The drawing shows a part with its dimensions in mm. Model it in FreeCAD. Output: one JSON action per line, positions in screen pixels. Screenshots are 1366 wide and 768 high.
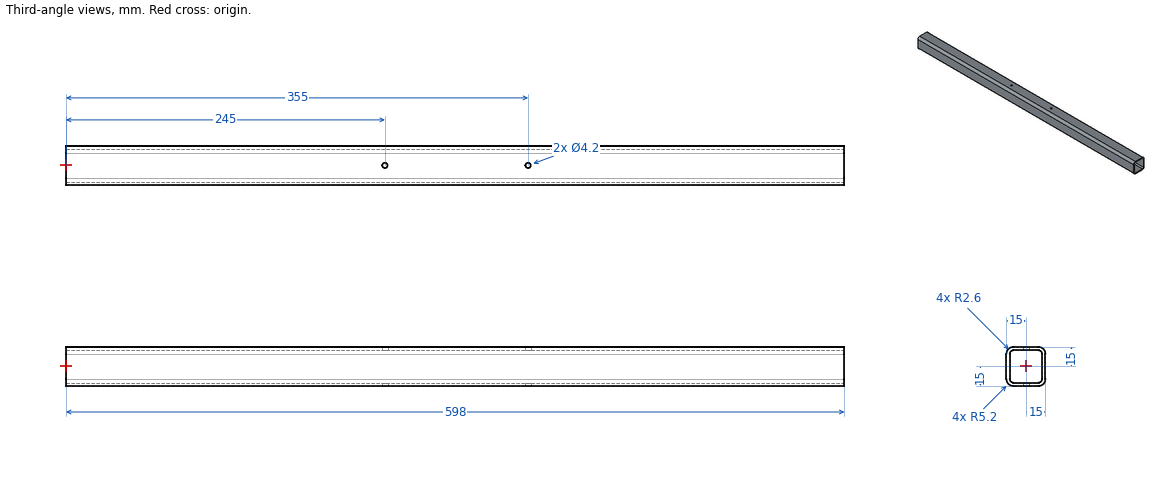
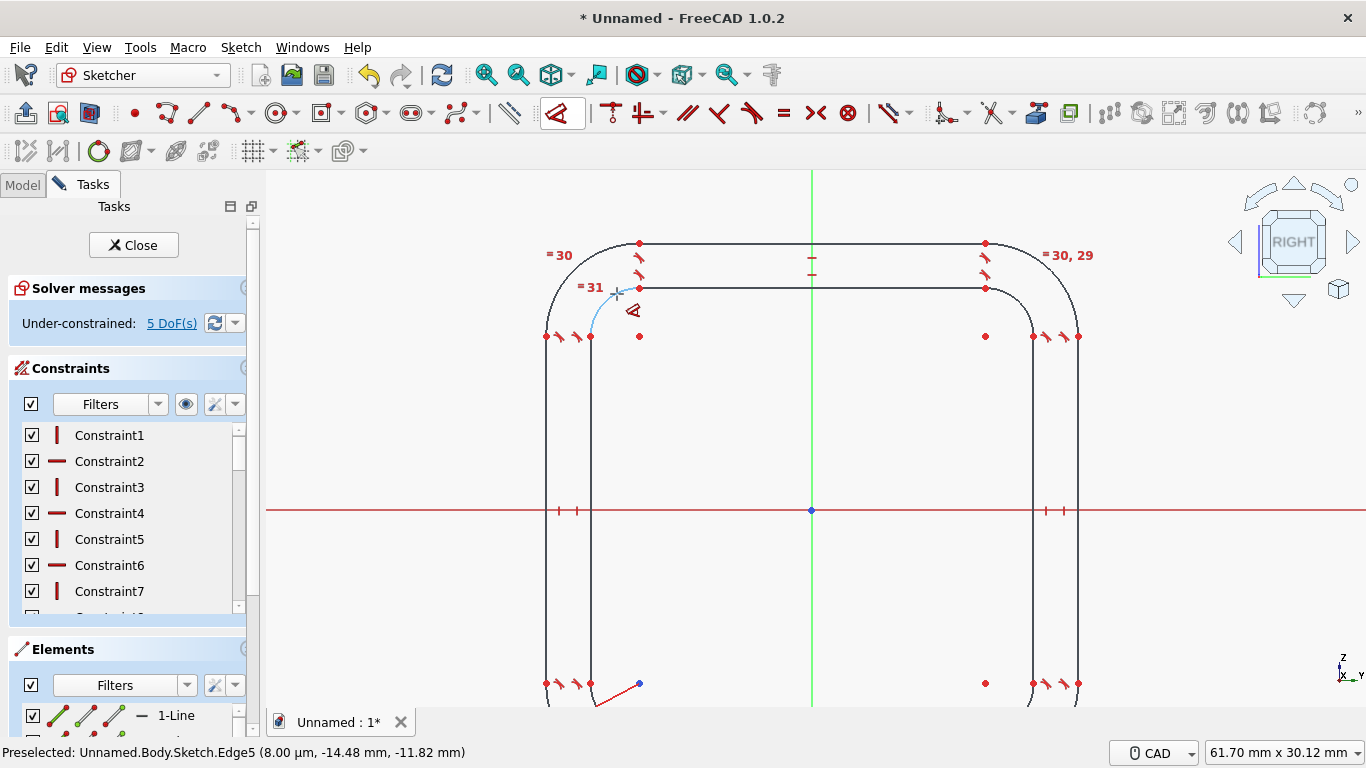
{"action": "left_click", "coordinate": [617, 293]}
{"action": "left_click", "coordinate": [680, 267]}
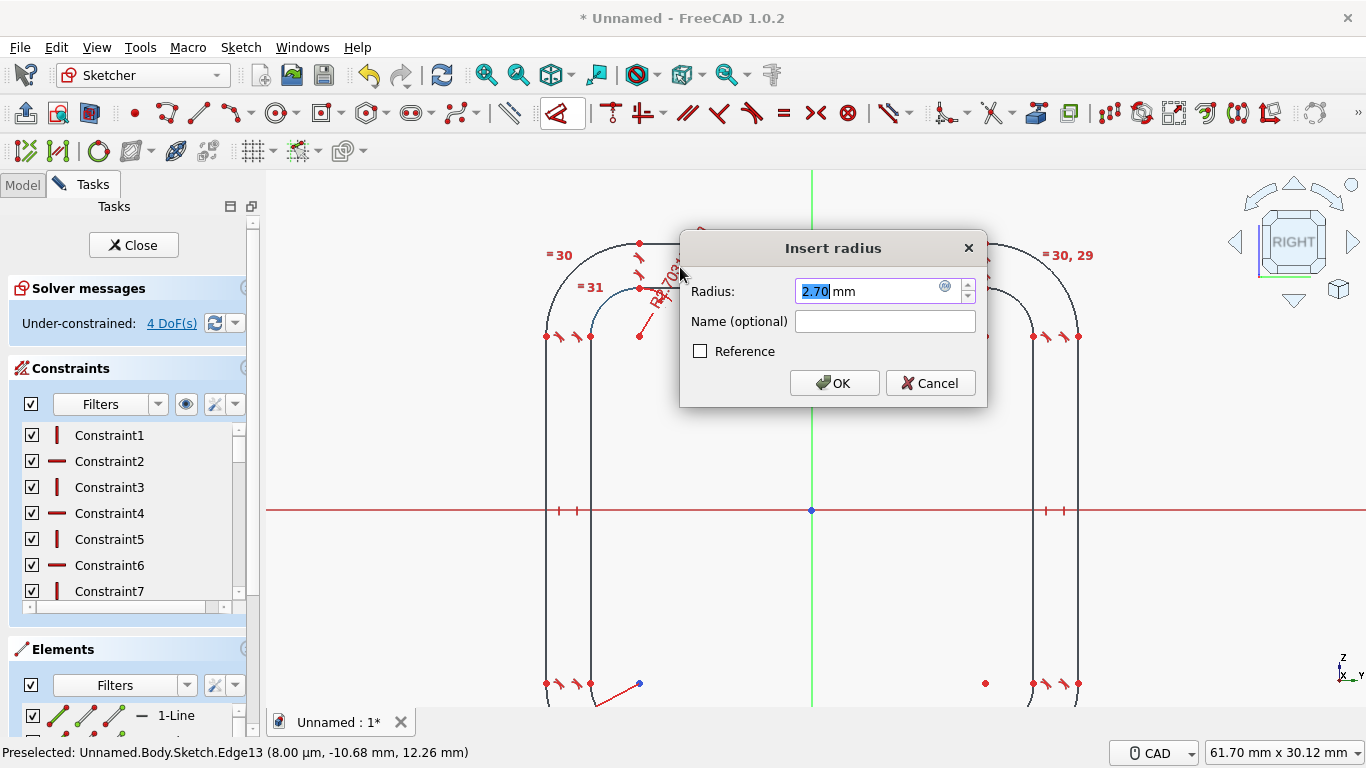
{"action": "type", "text": "2.6"}
{"action": "key", "text": "Return"}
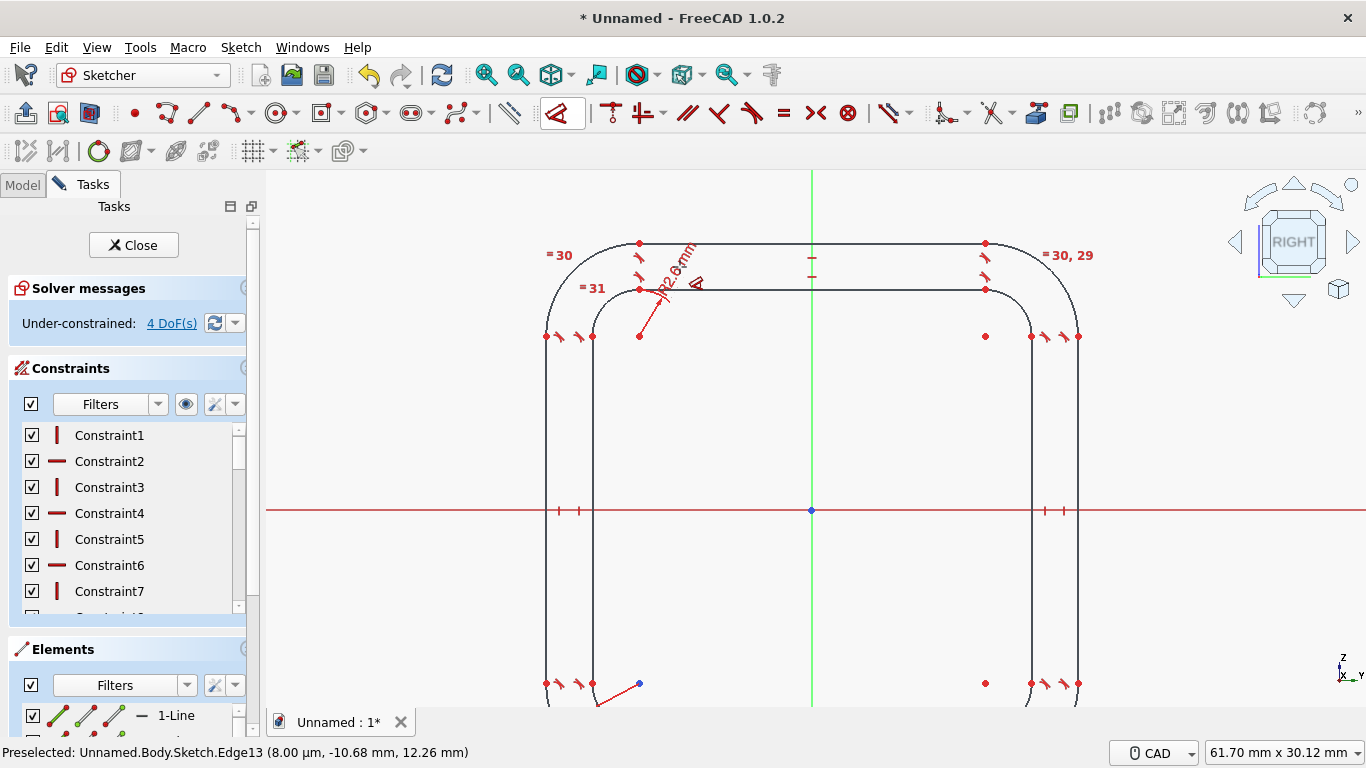
{"action": "left_click", "coordinate": [546, 336]}
{"action": "left_click", "coordinate": [586, 302]}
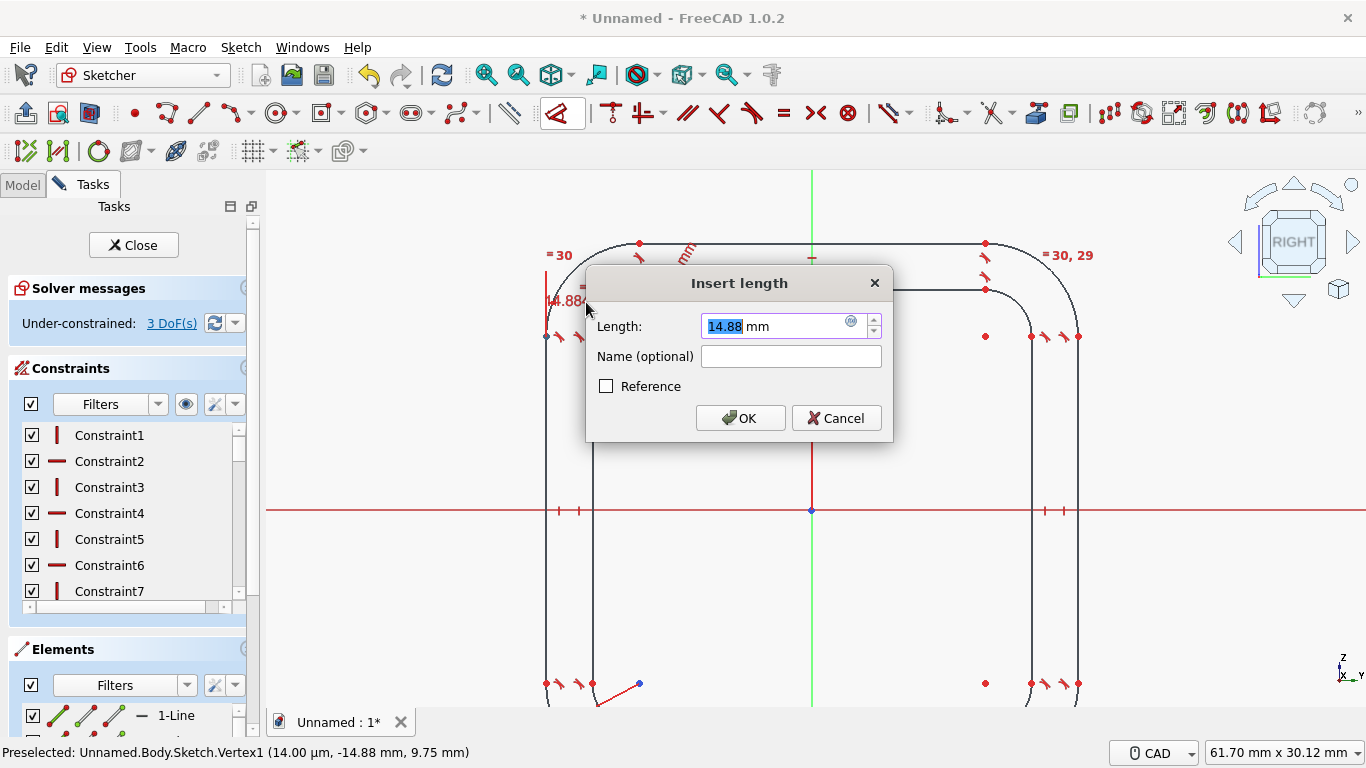
{"action": "type", "text": "15"}
{"action": "key", "text": "Return"}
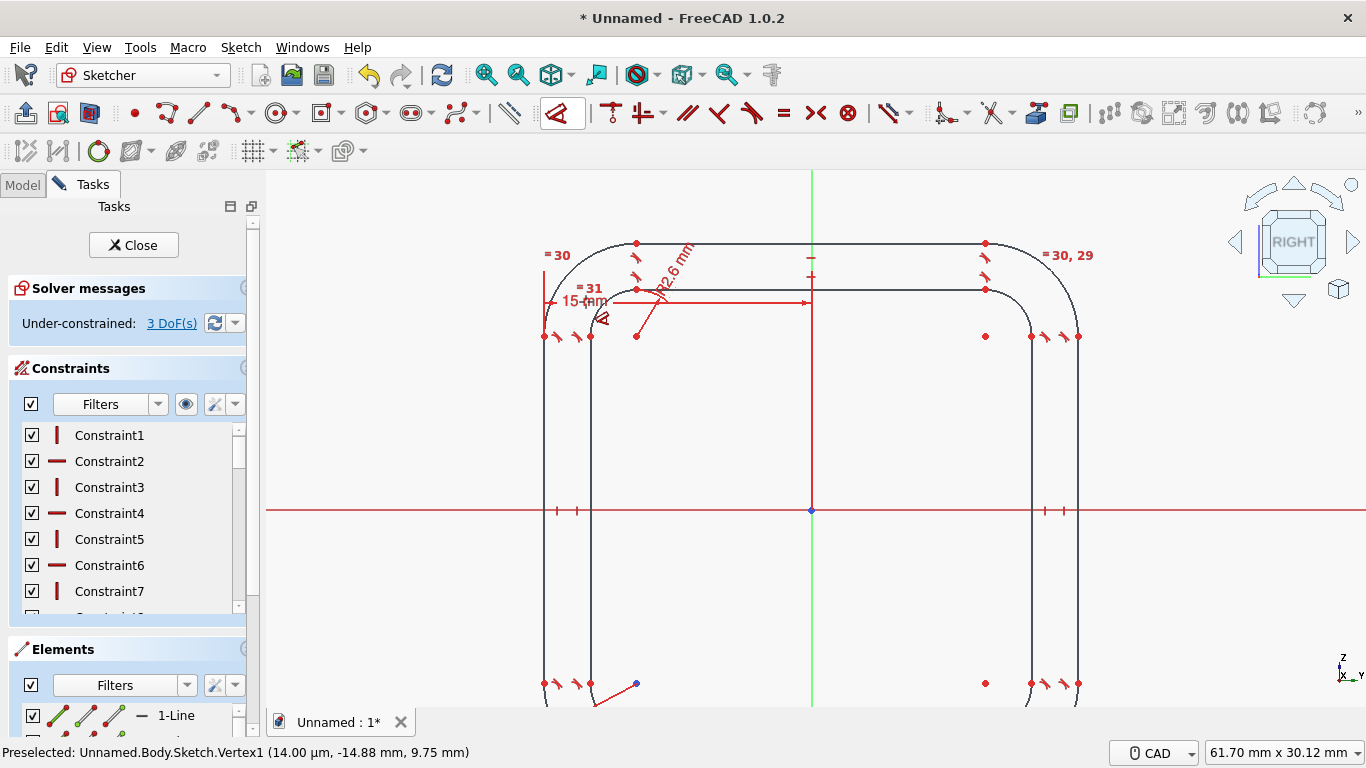
{"action": "scroll", "coordinate": [617, 293], "scroll_direction": "down", "scroll_amount": 2}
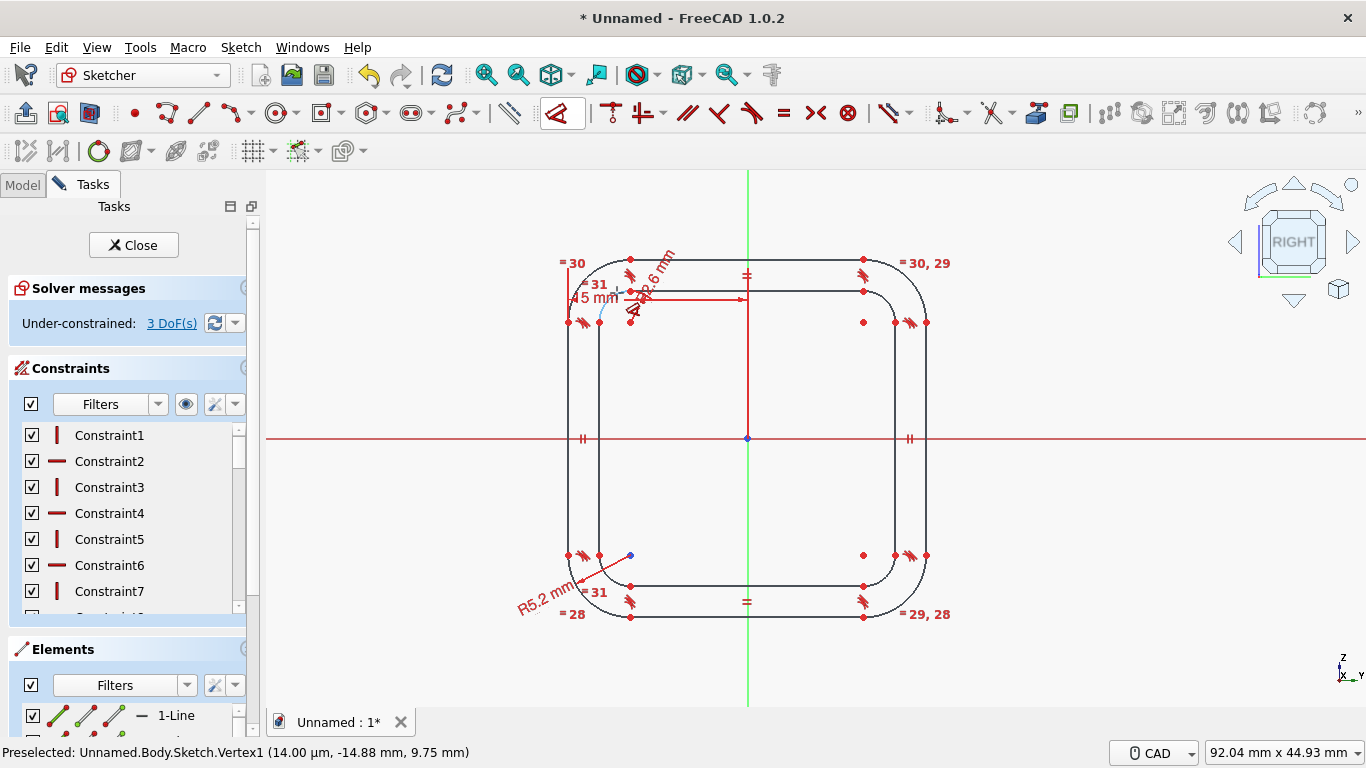
{"action": "left_click", "coordinate": [630, 617]}
{"action": "left_click", "coordinate": [782, 528]}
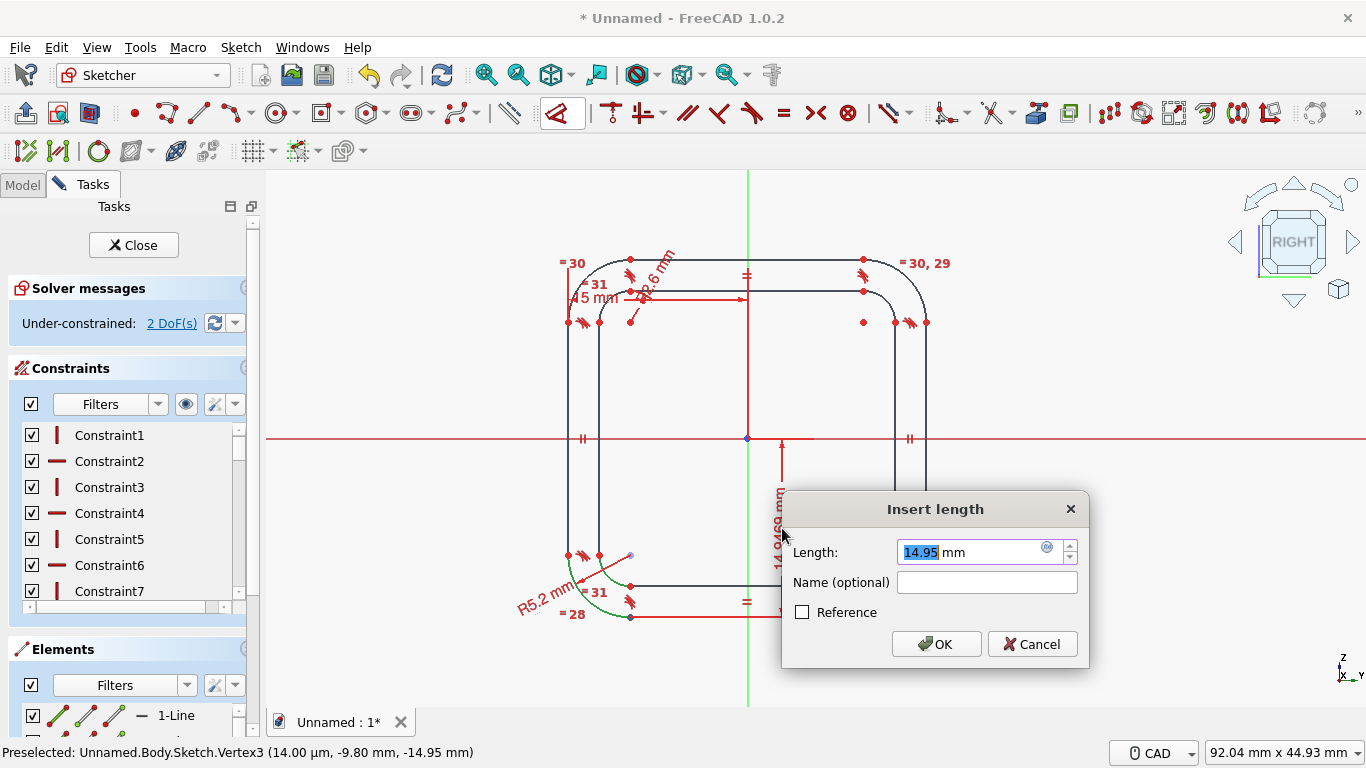
{"action": "type", "text": "15"}
{"action": "key", "text": "Return"}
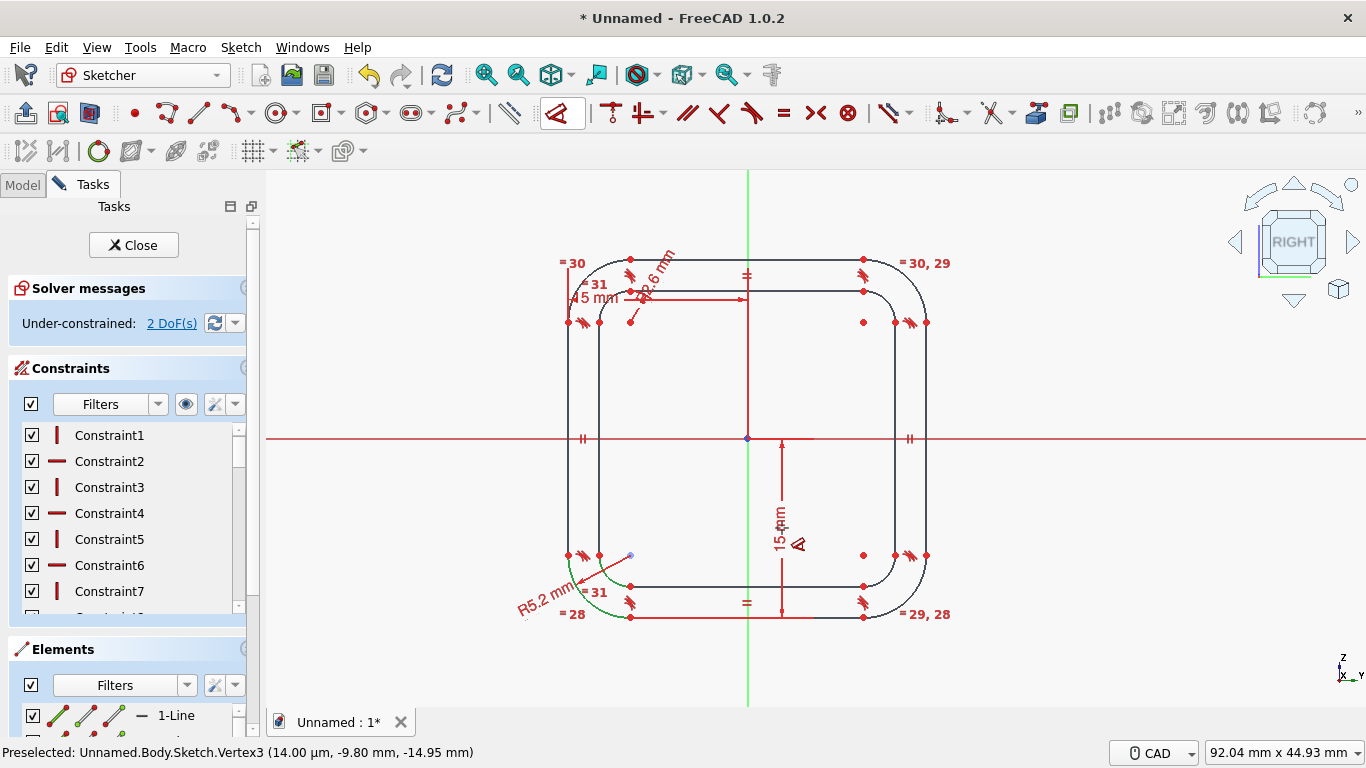
{"action": "left_click", "coordinate": [926, 556]}
{"action": "left_click", "coordinate": [899, 590]}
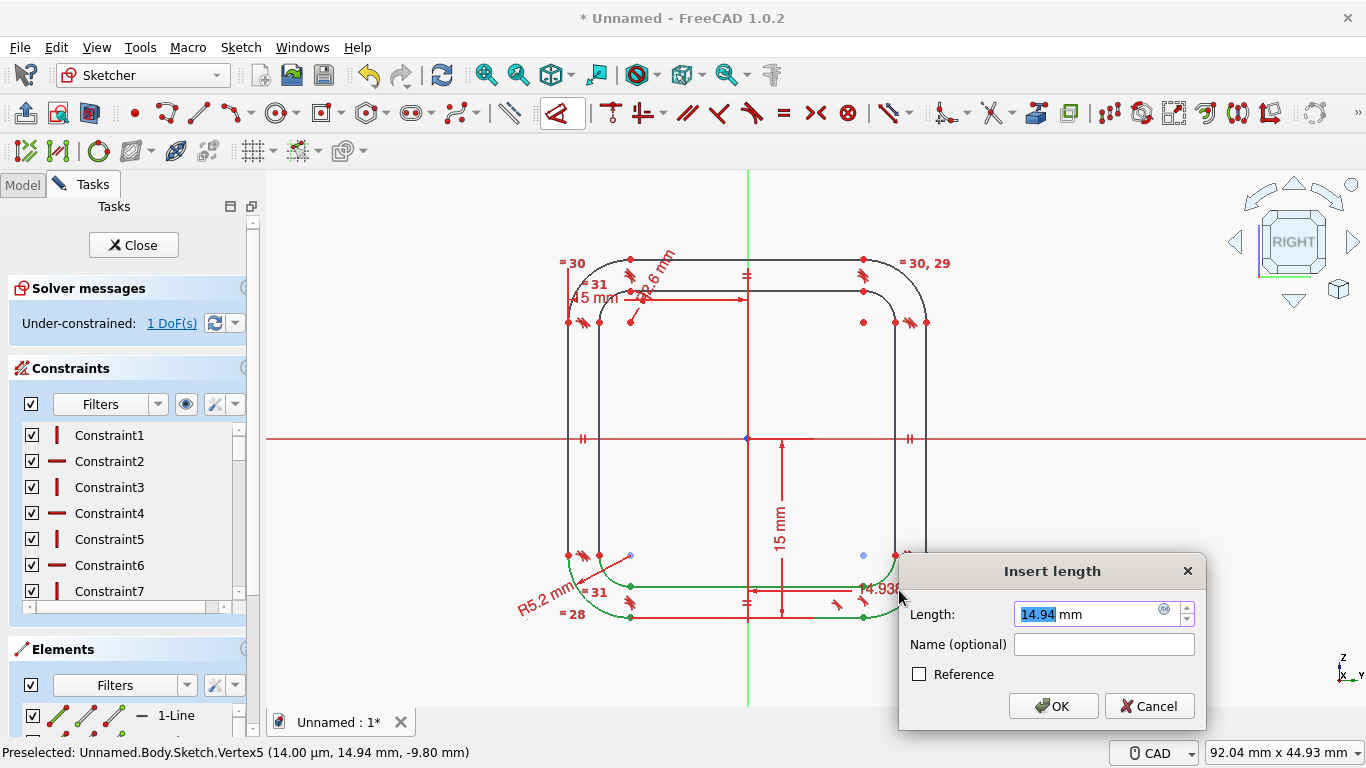
{"action": "type", "text": "15"}
{"action": "key", "text": "Return"}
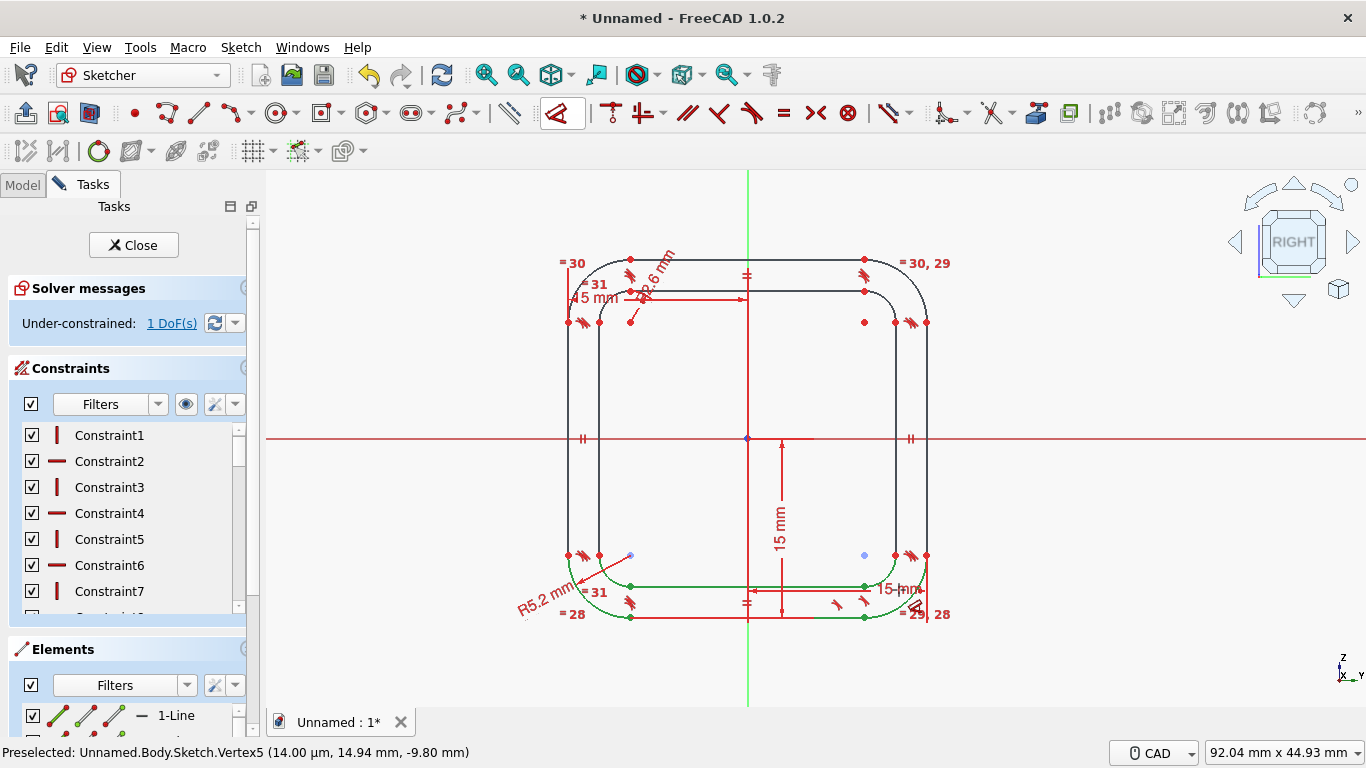
{"action": "left_click", "coordinate": [865, 260]}
{"action": "left_click", "coordinate": [899, 287]}